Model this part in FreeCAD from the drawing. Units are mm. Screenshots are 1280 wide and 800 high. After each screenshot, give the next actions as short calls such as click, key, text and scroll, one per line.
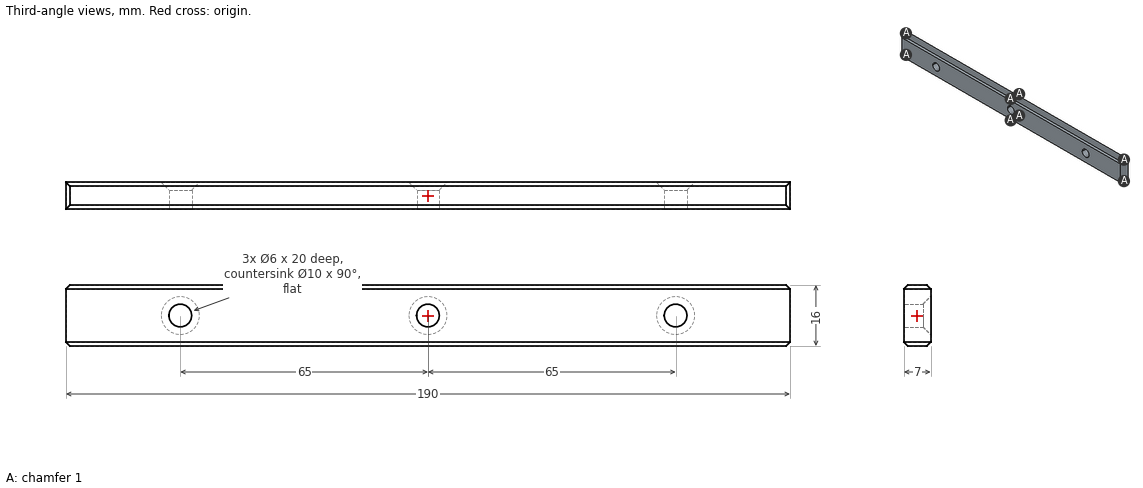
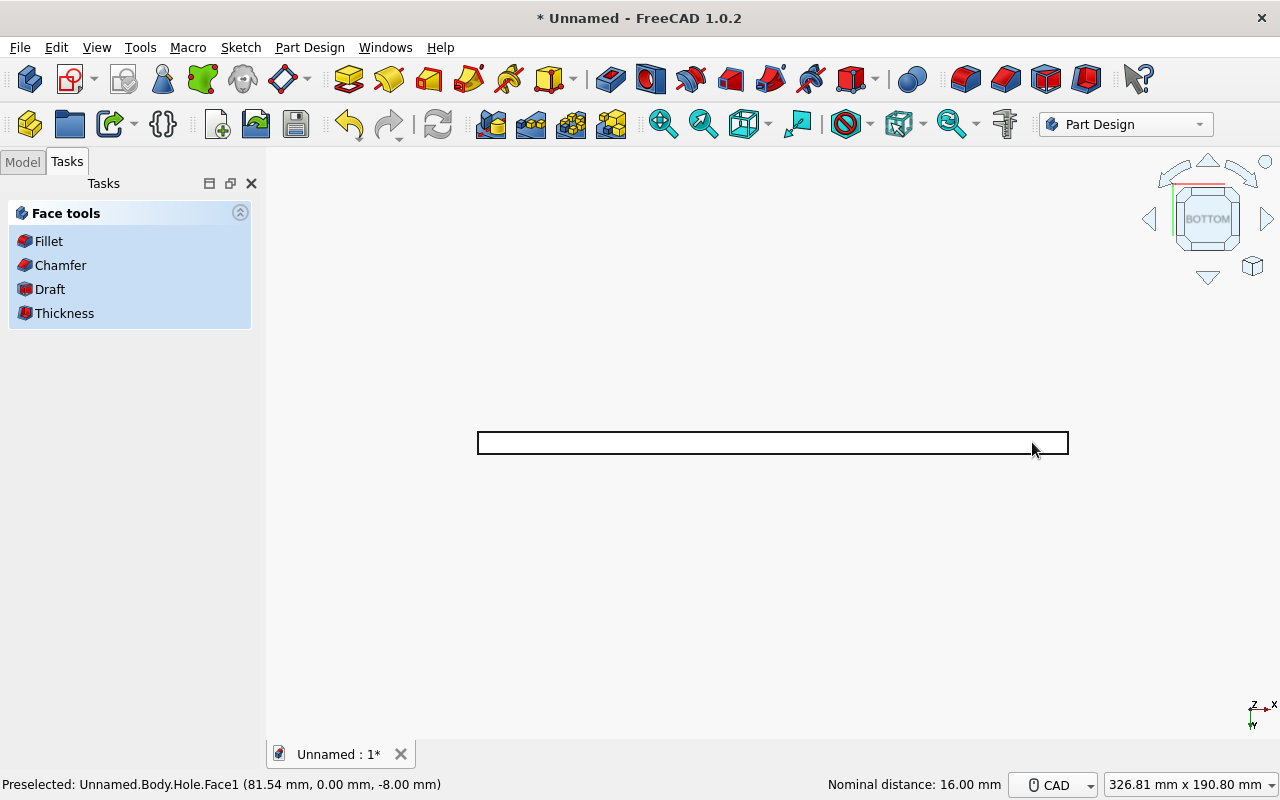
click(1006, 80)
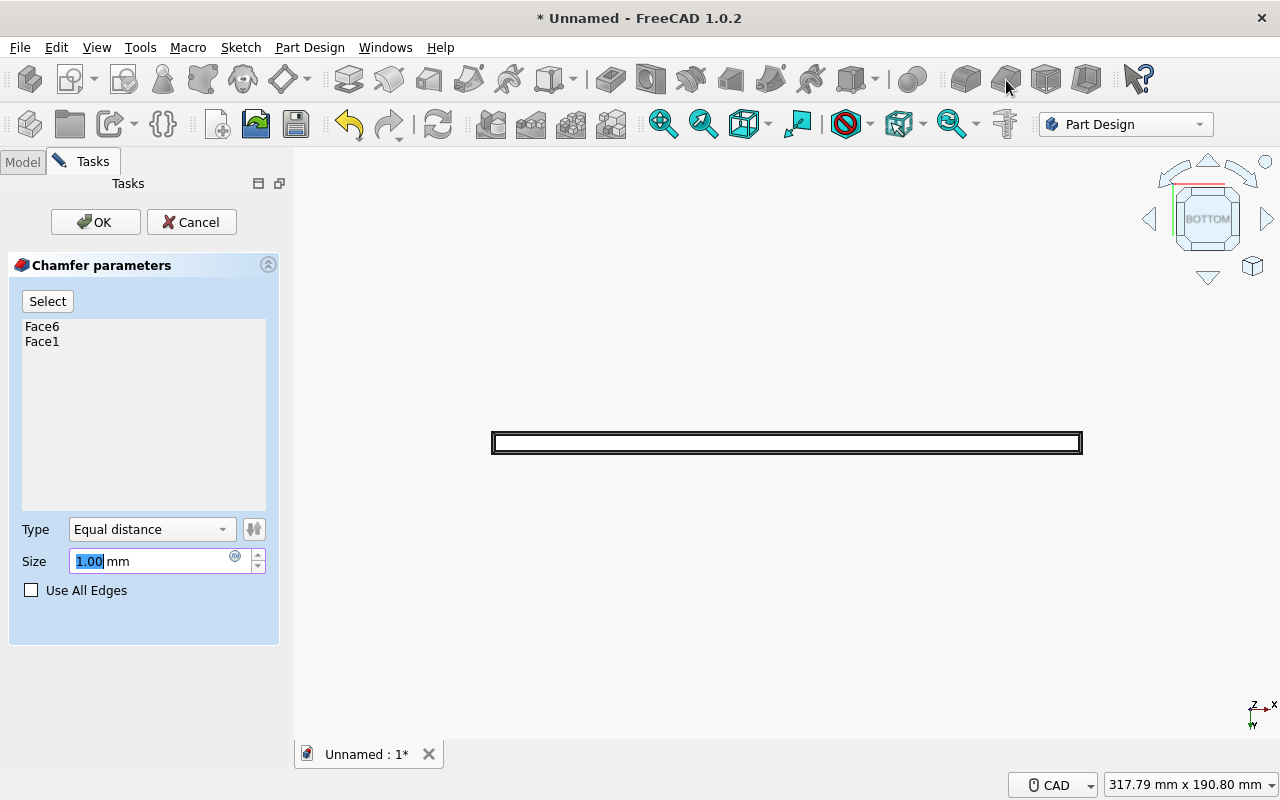
text(1)
key(Tab)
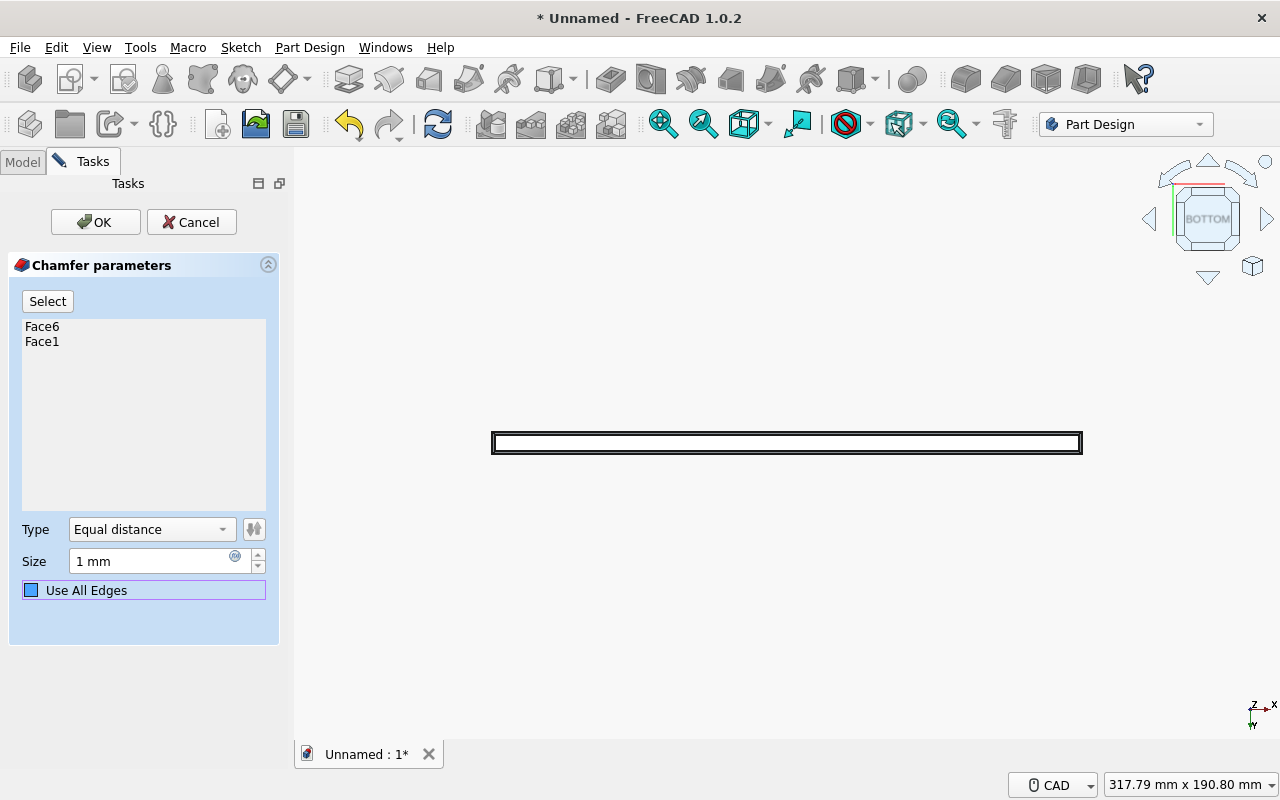
click(96, 222)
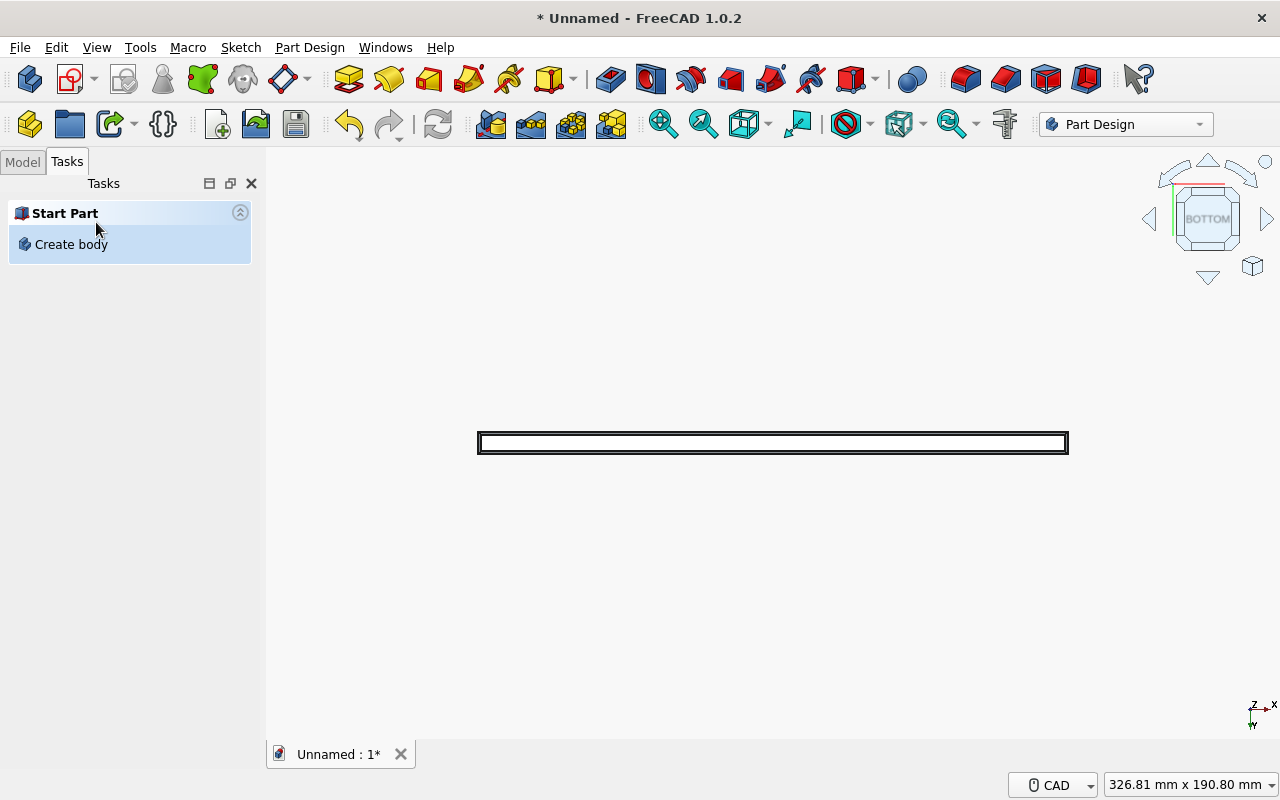
key(0)